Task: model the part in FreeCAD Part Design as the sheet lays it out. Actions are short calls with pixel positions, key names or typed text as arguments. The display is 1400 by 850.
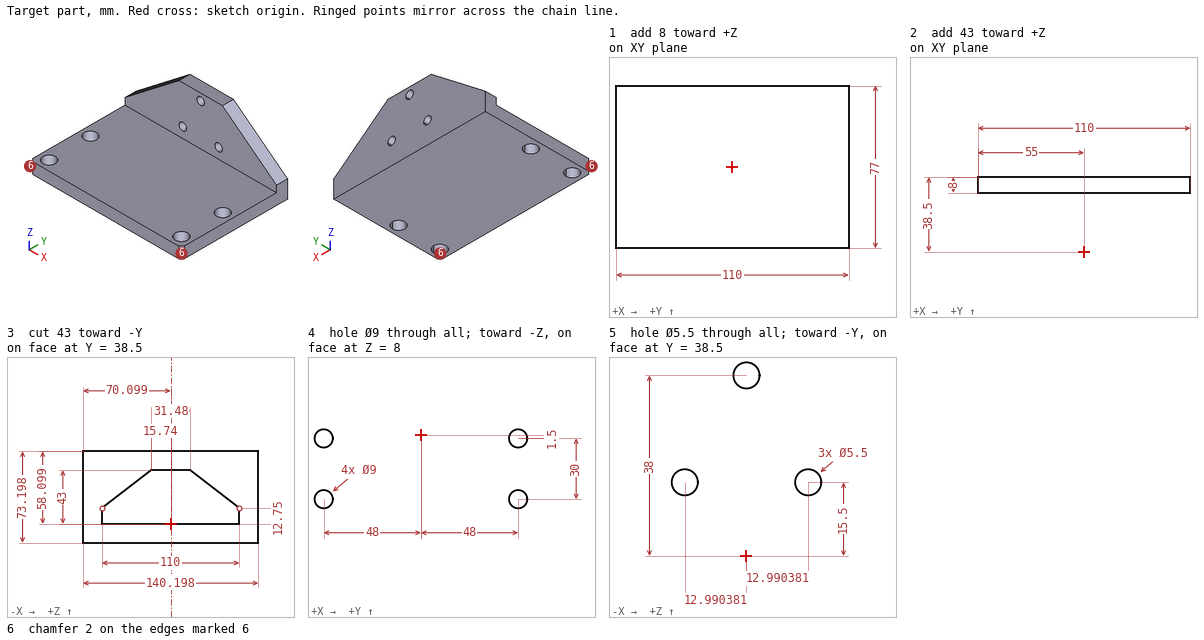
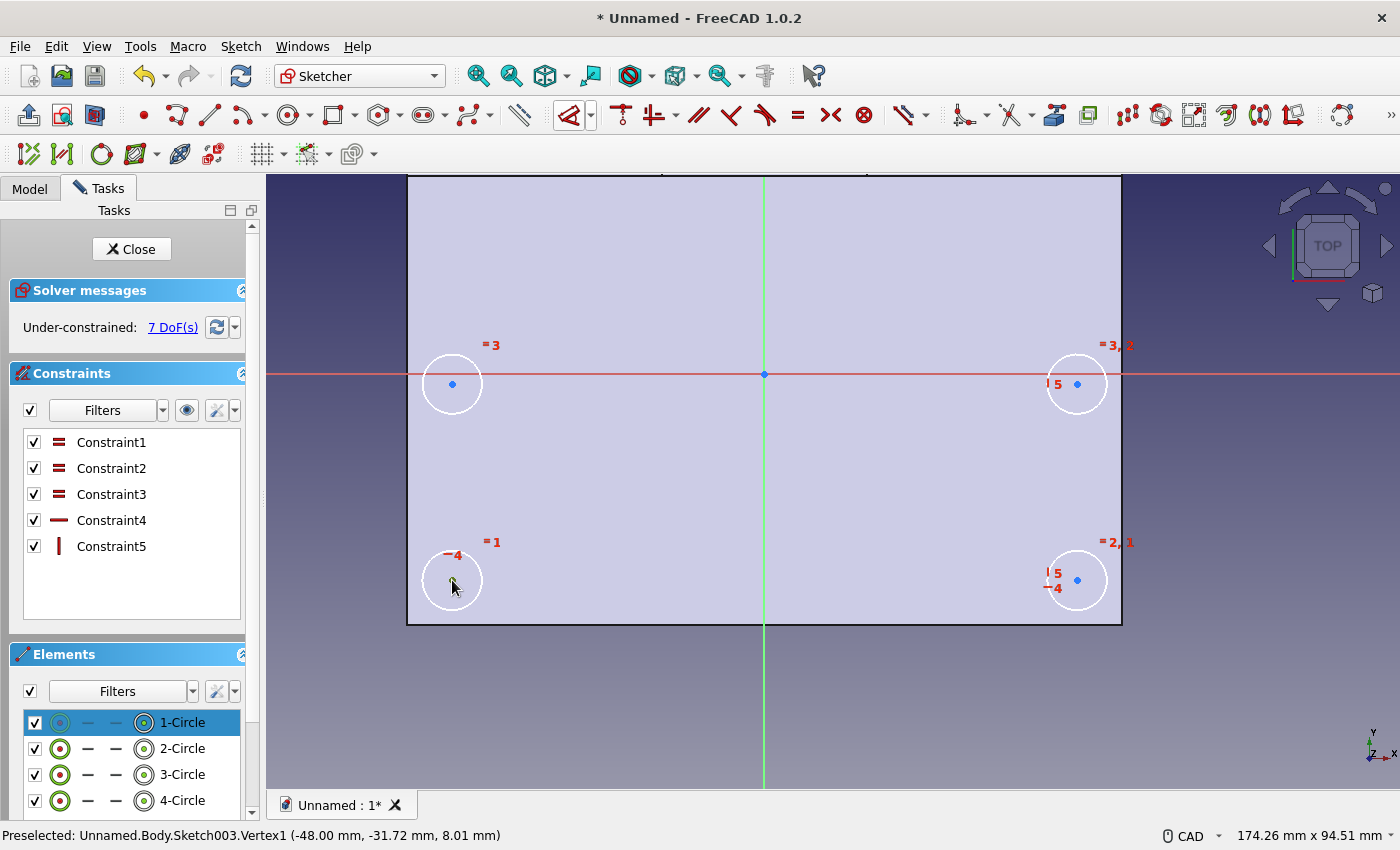
click(452, 384)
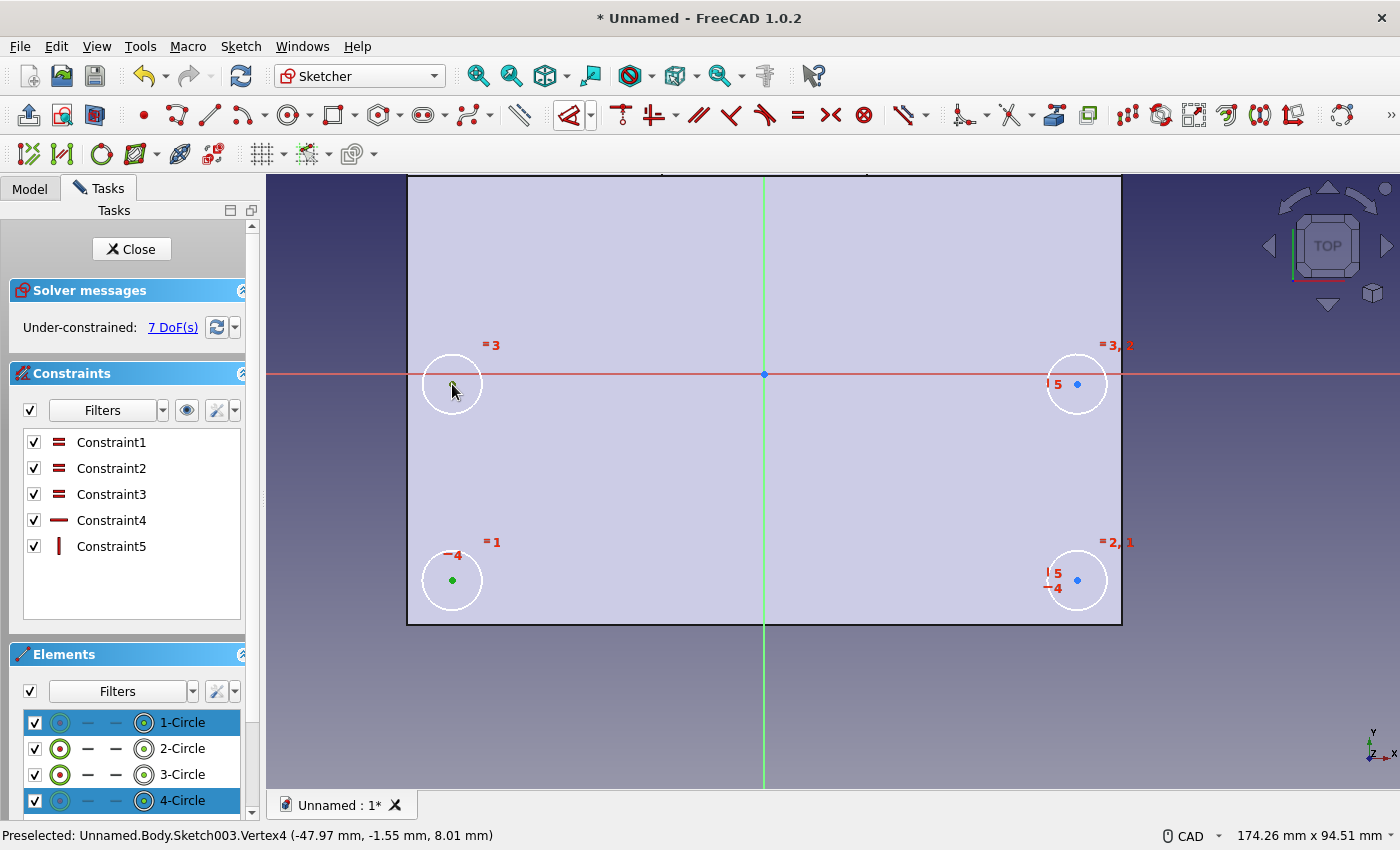
key(v)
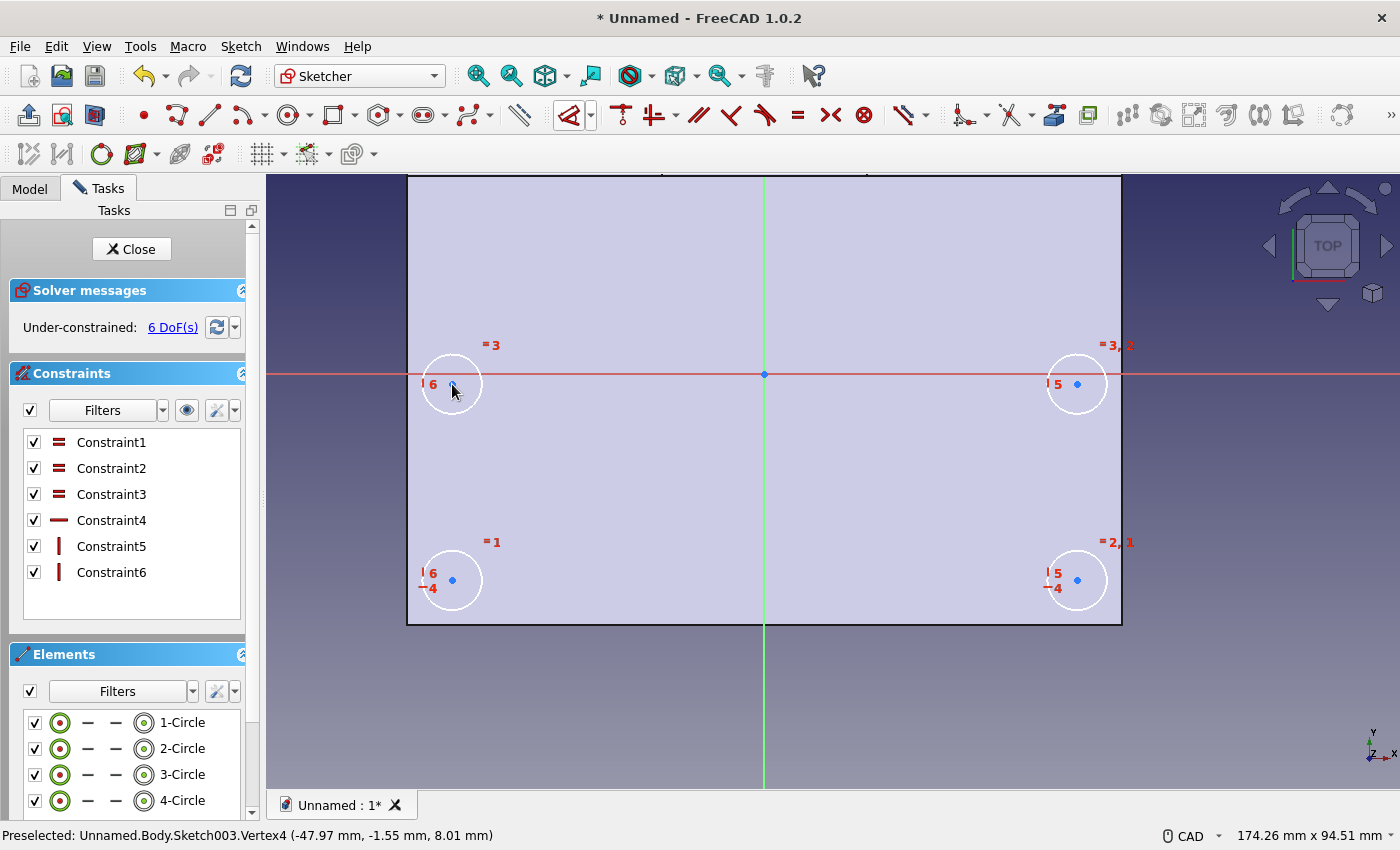
click(1077, 384)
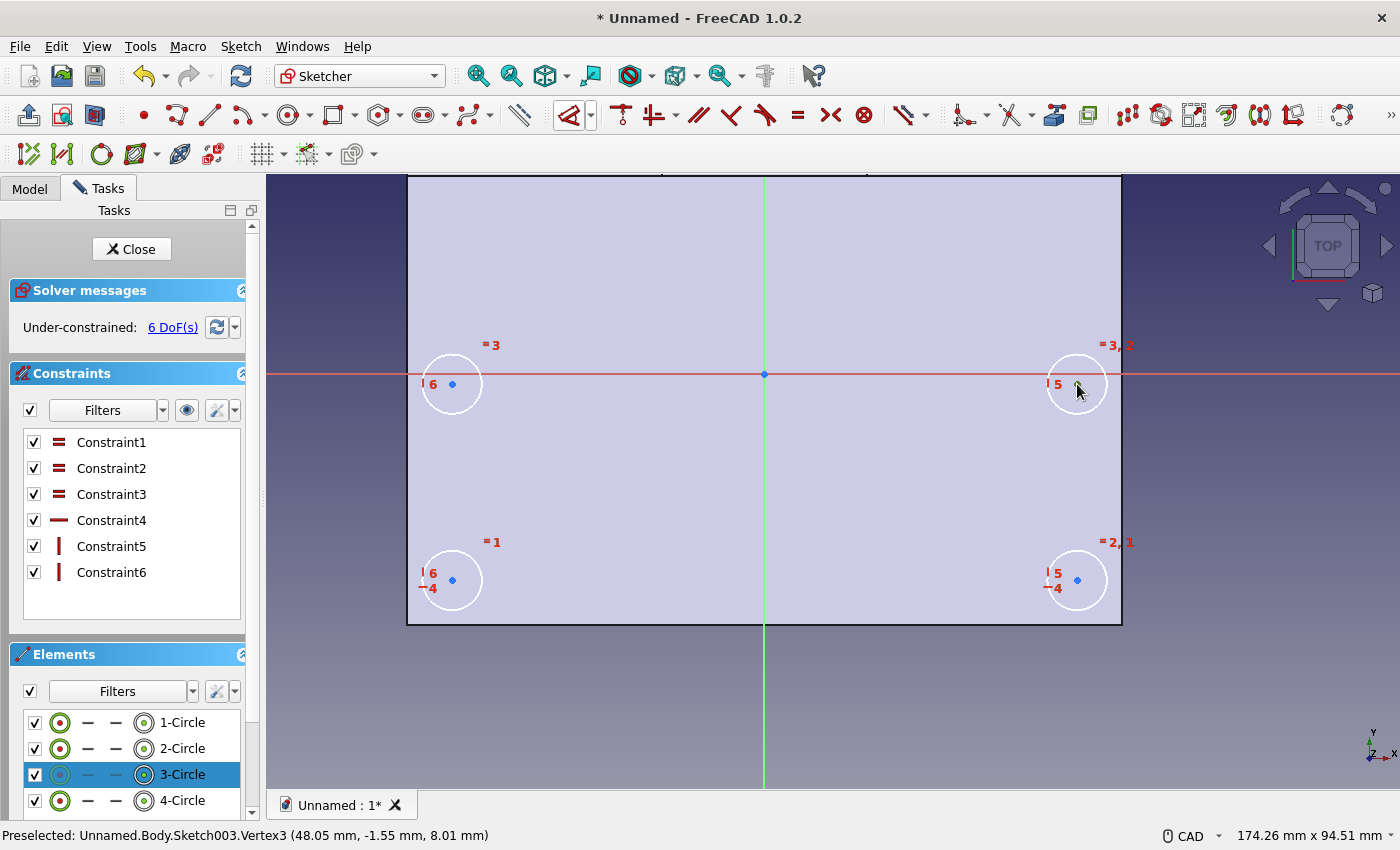
click(452, 384)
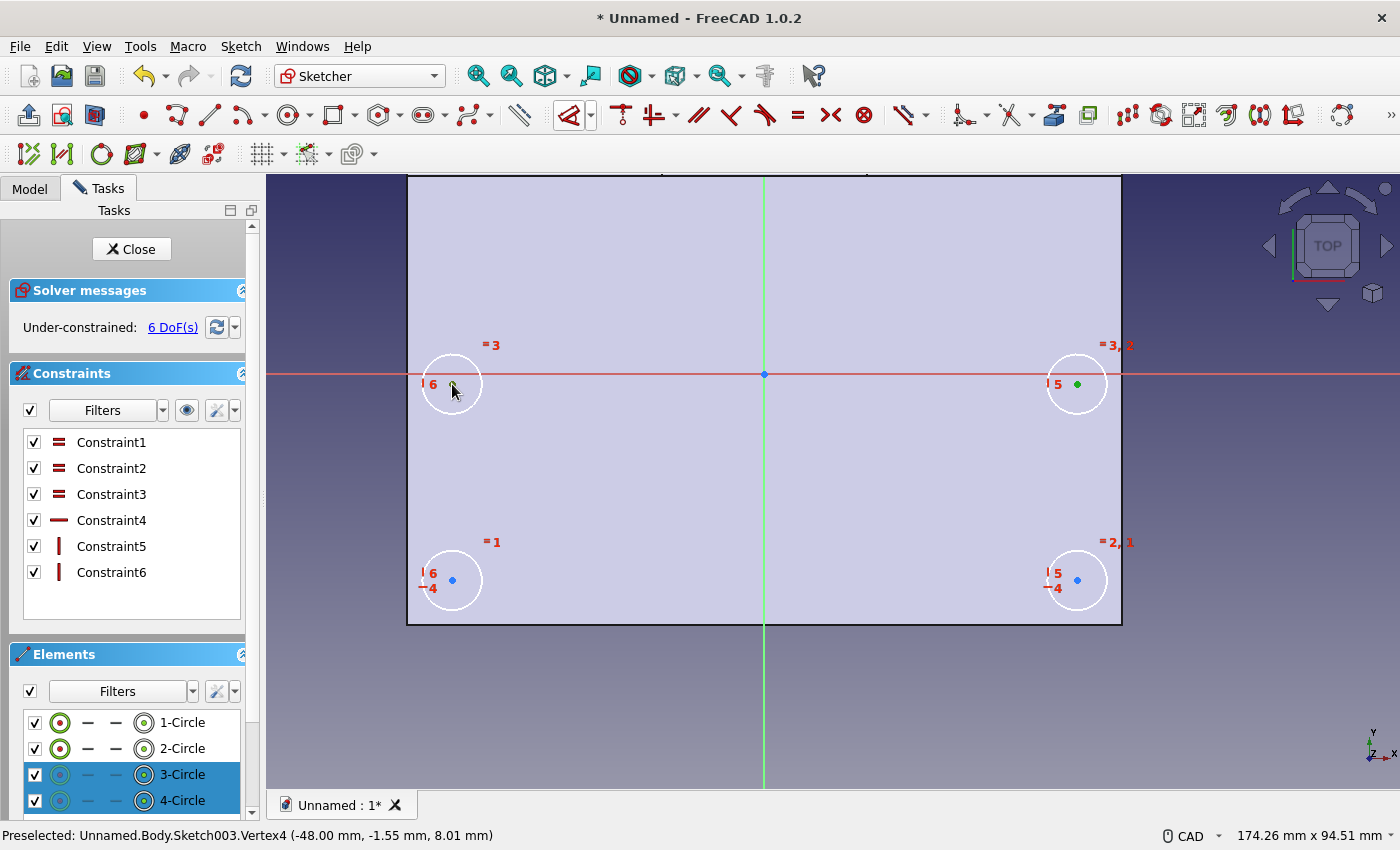
click(676, 116)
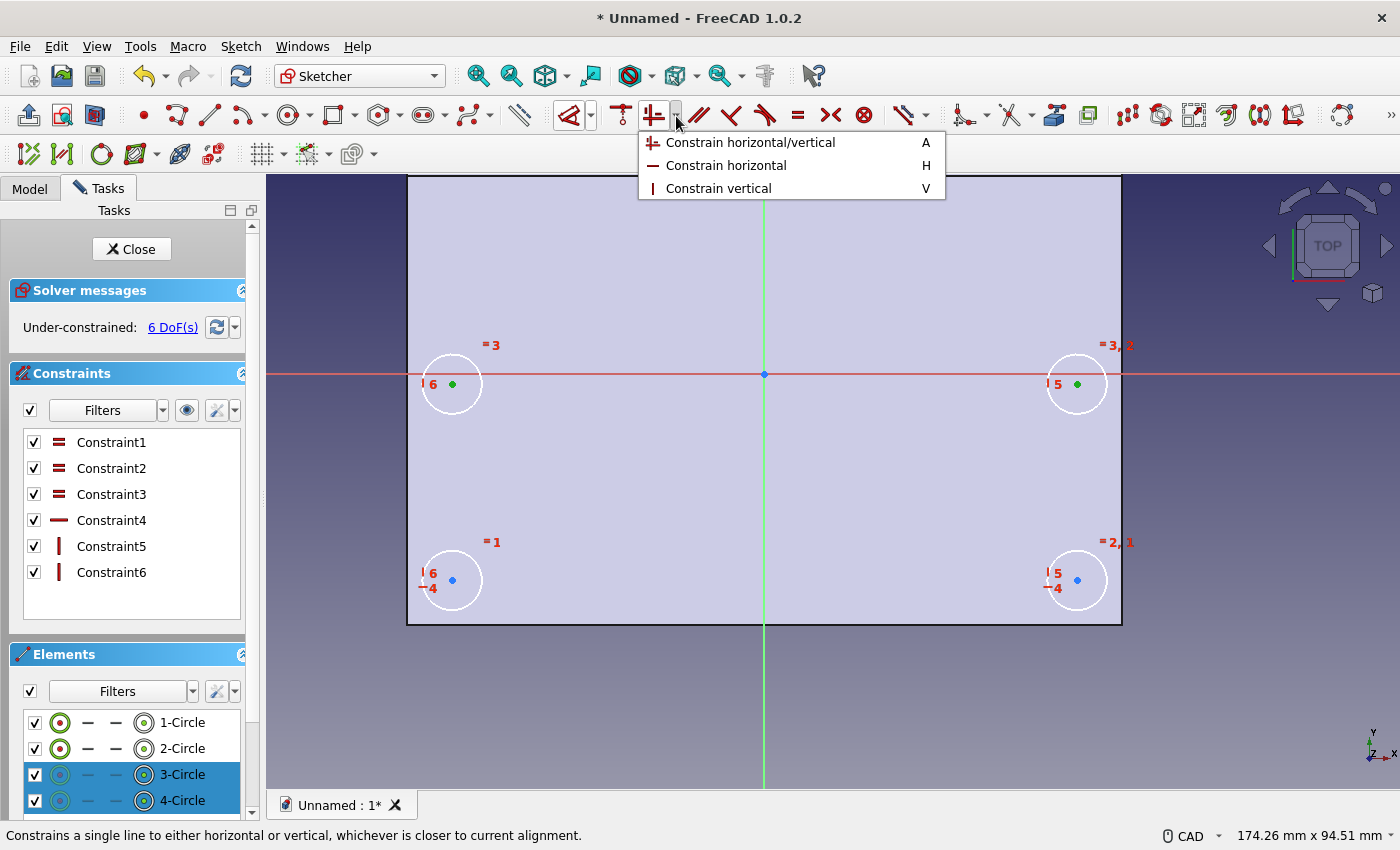
click(792, 166)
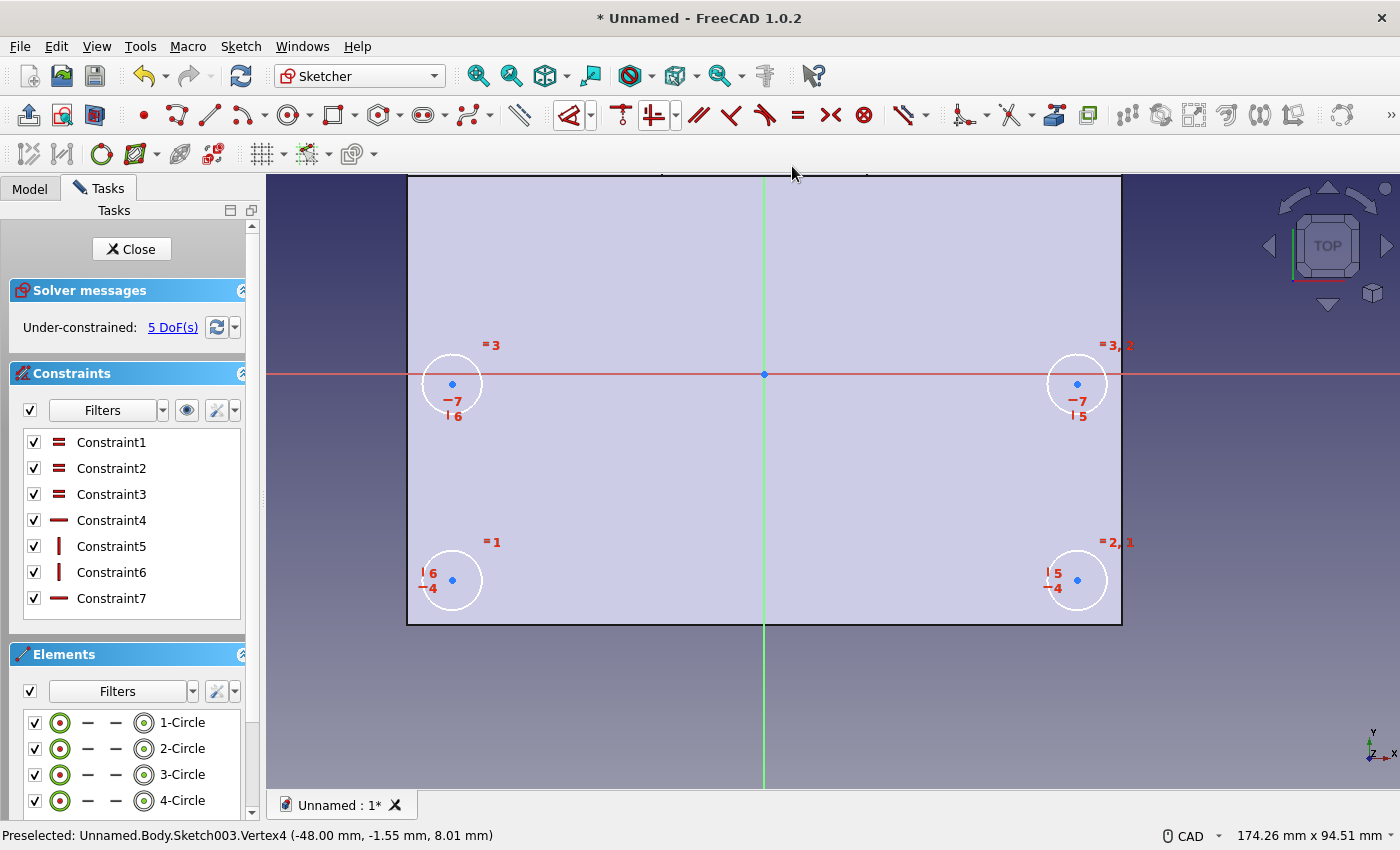
click(473, 559)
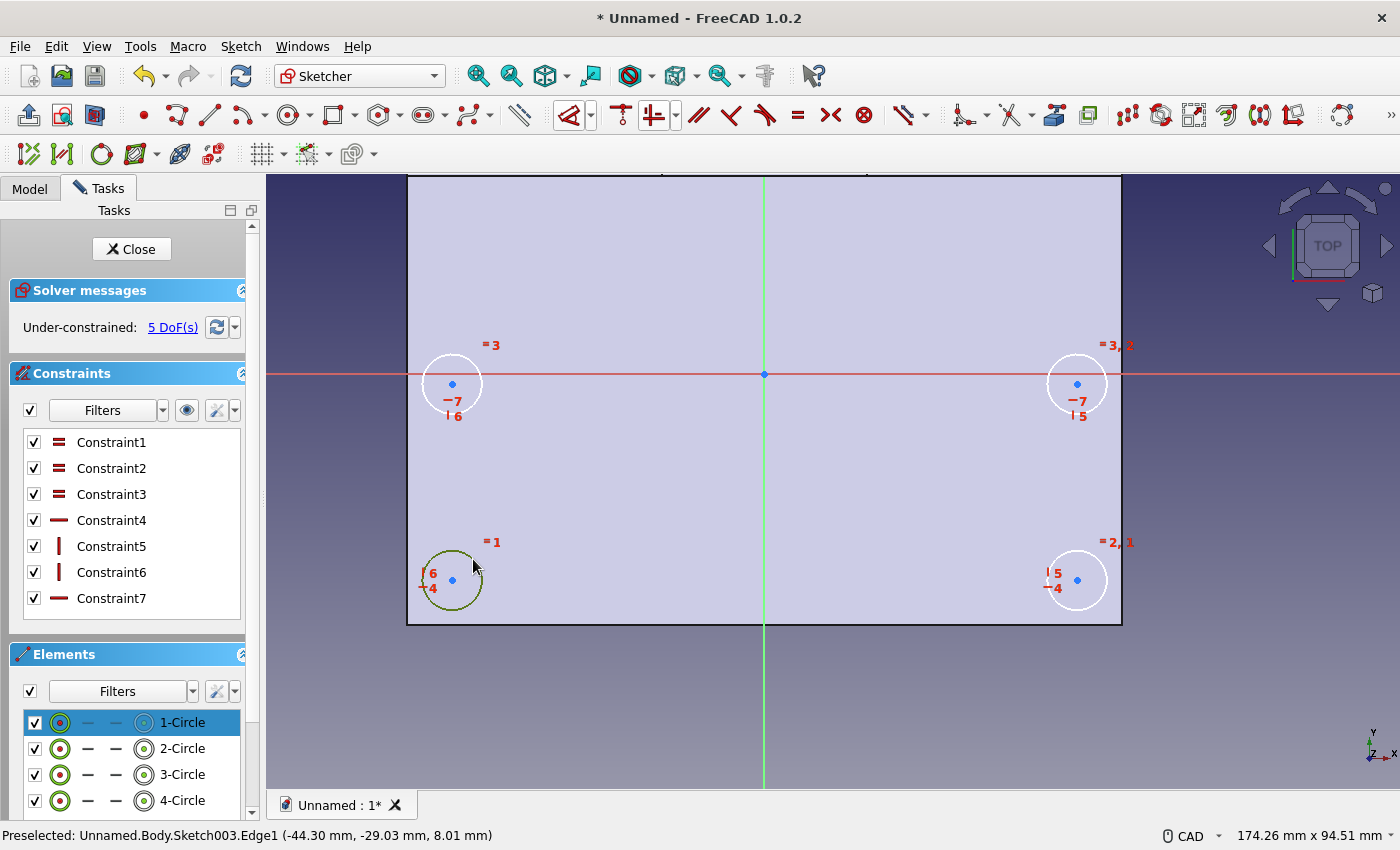
key(k)
key(o)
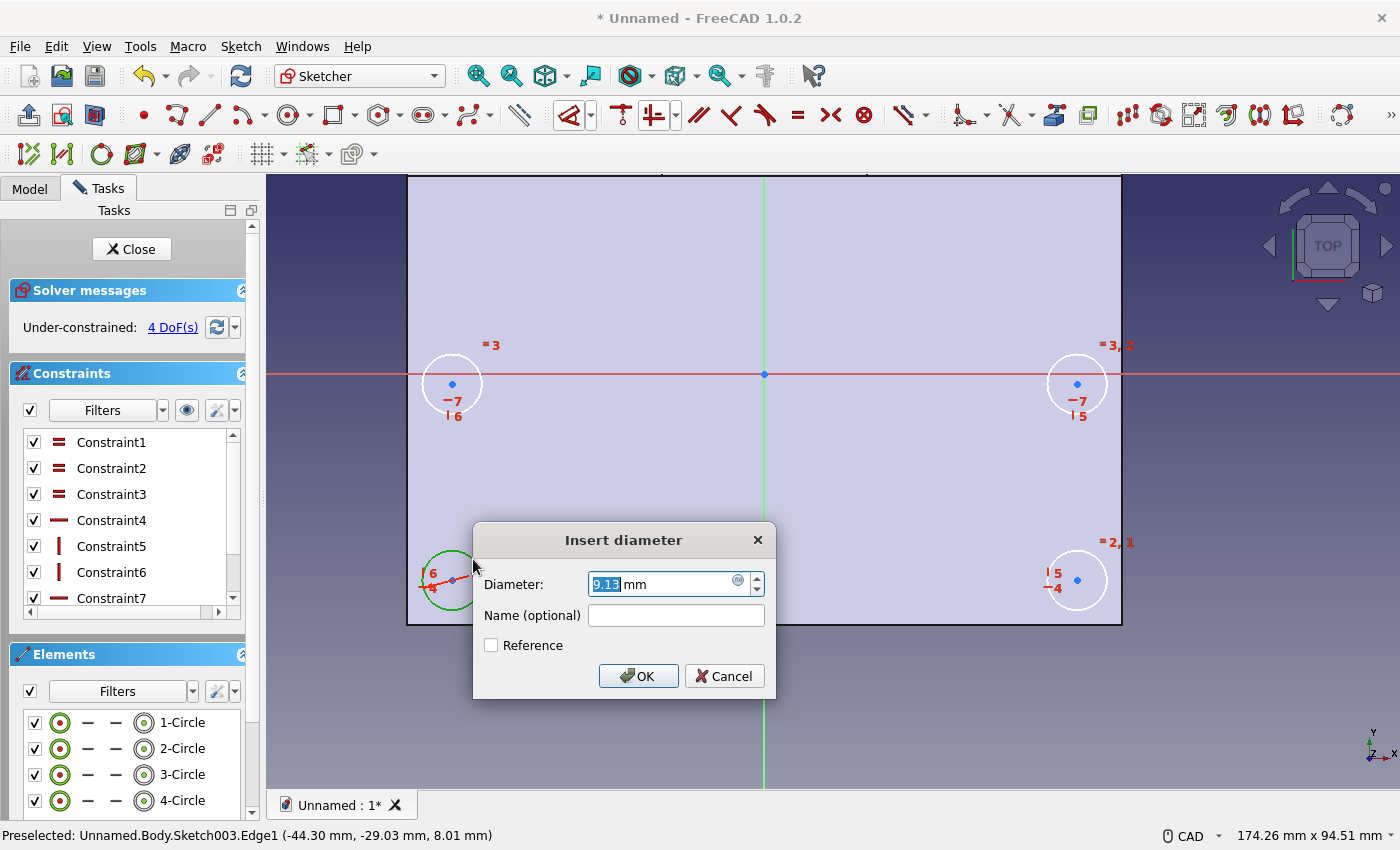
text(9)
key(Return)